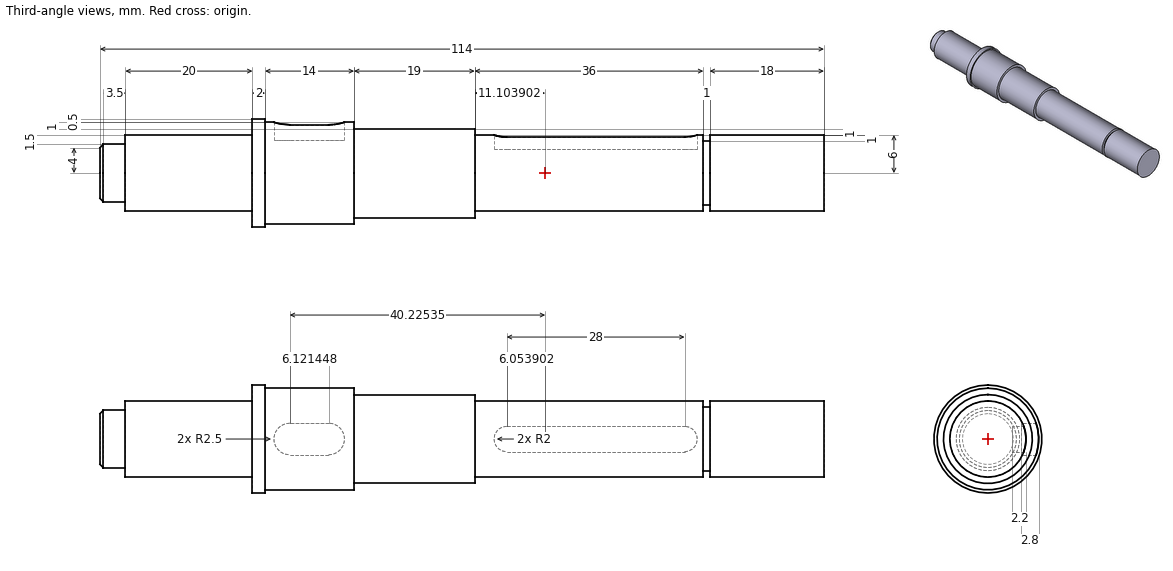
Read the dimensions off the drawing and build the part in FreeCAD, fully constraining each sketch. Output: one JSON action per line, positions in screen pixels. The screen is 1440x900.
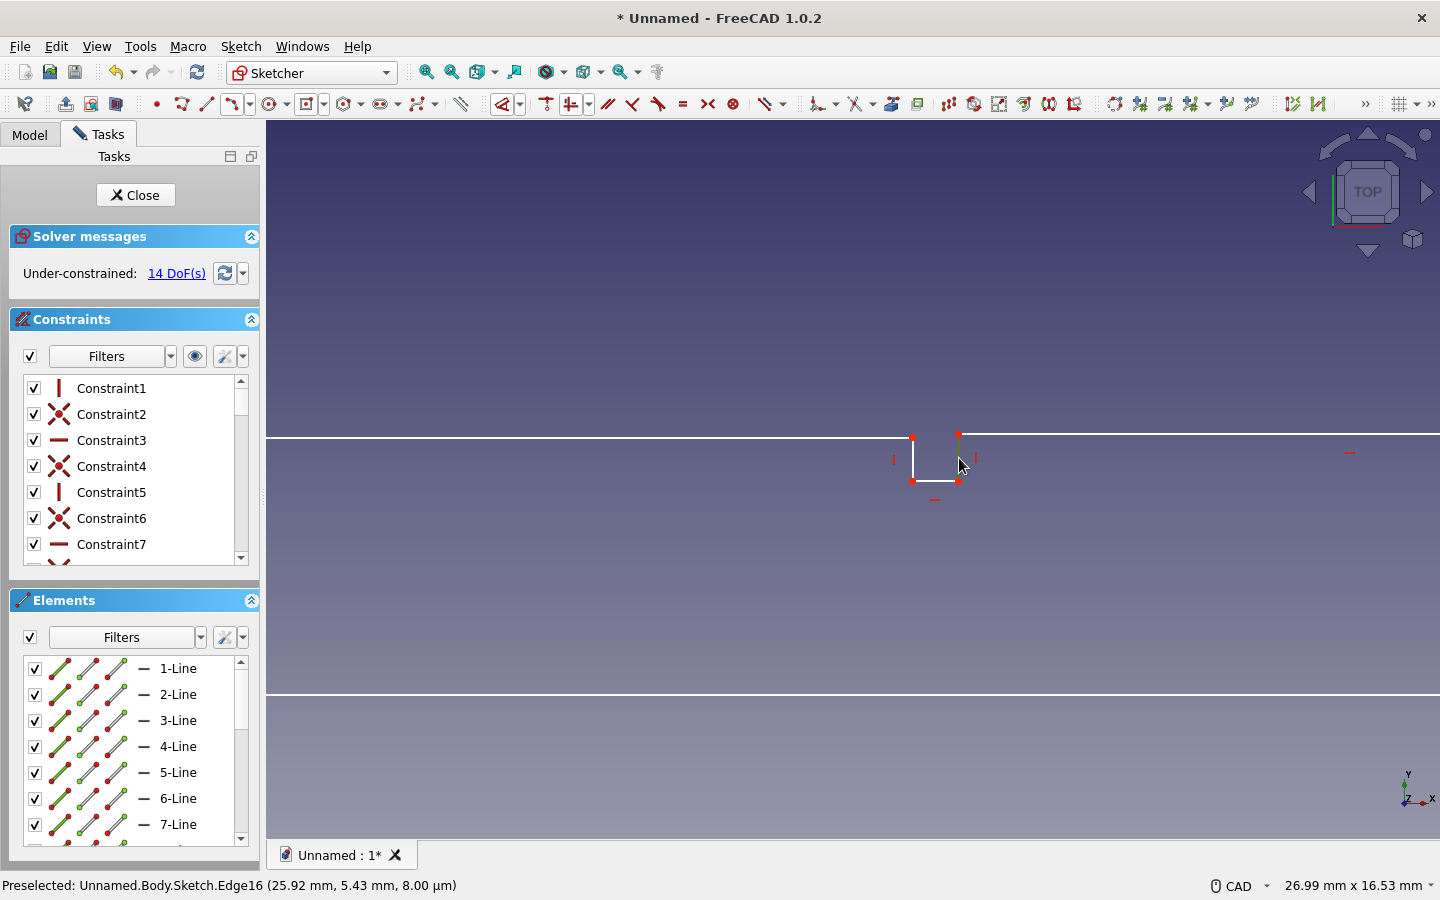
{"action": "left_click", "coordinate": [520, 104]}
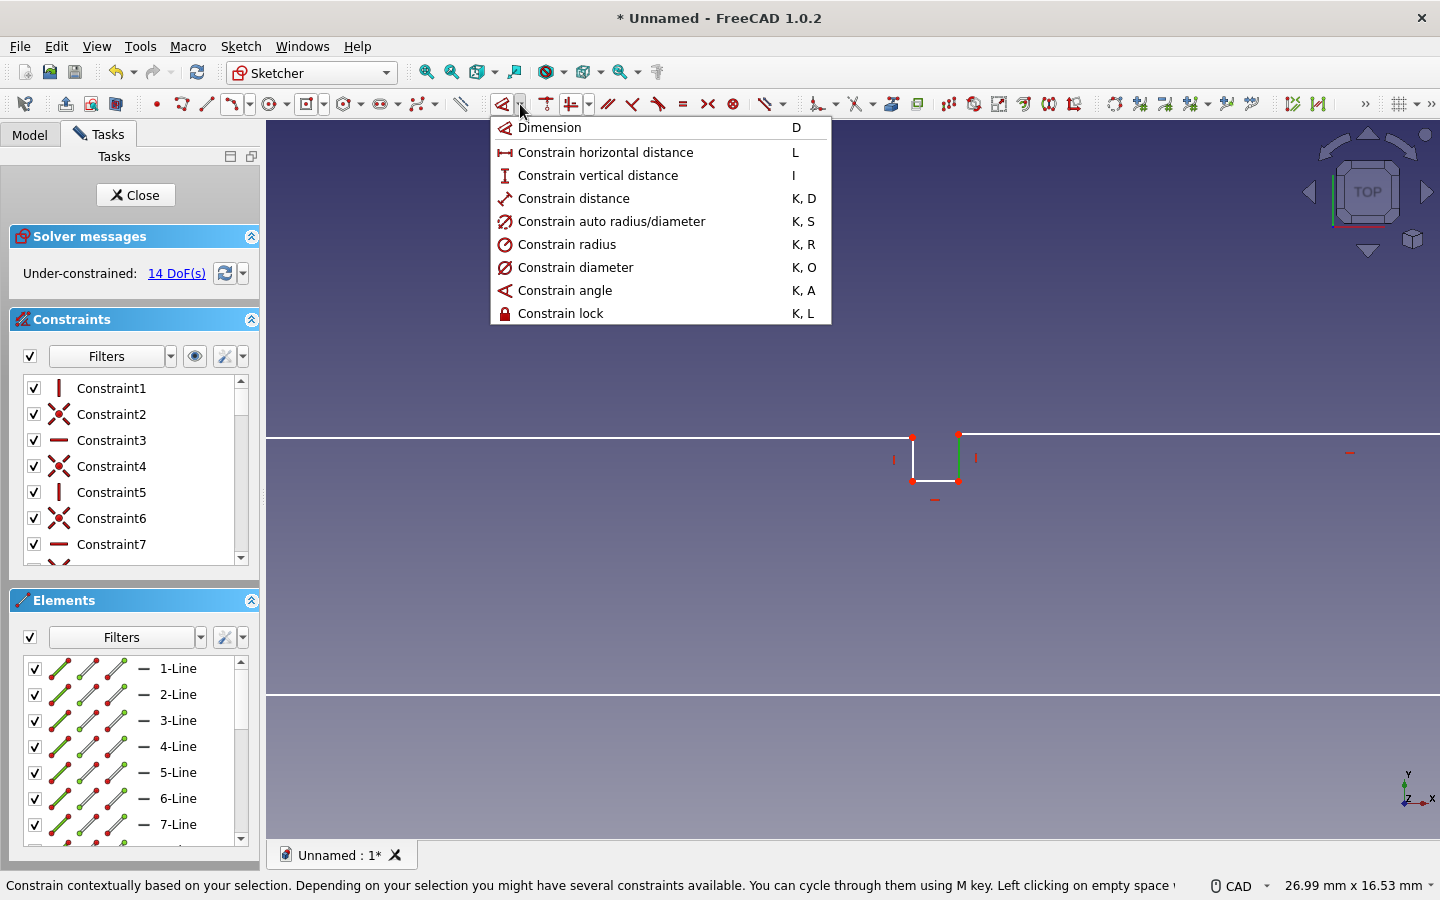
{"action": "left_click", "coordinate": [661, 176]}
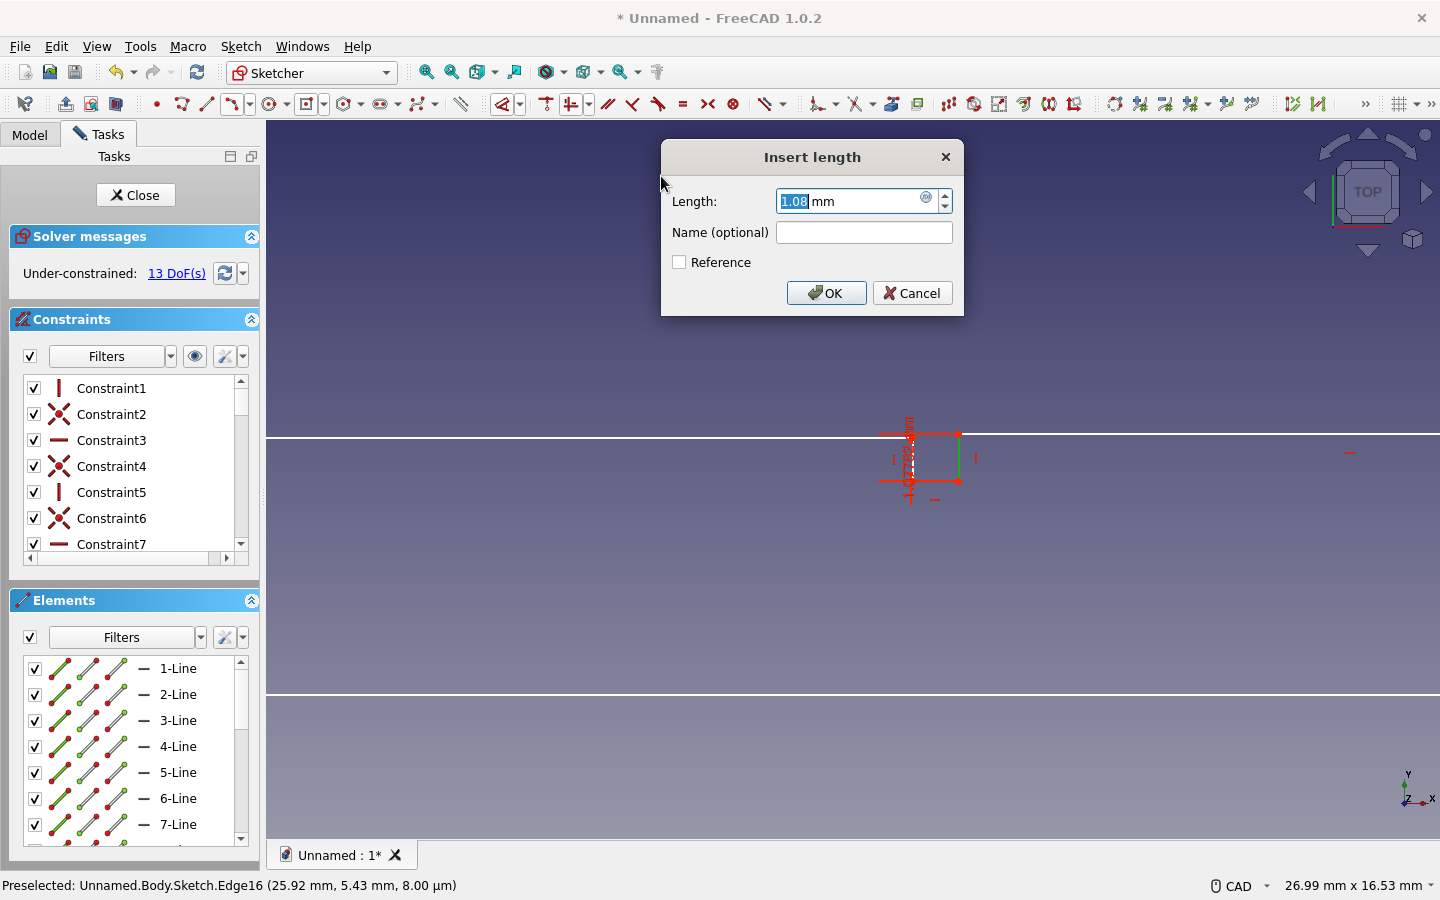
{"action": "type", "text": "1"}
{"action": "key", "text": "Return"}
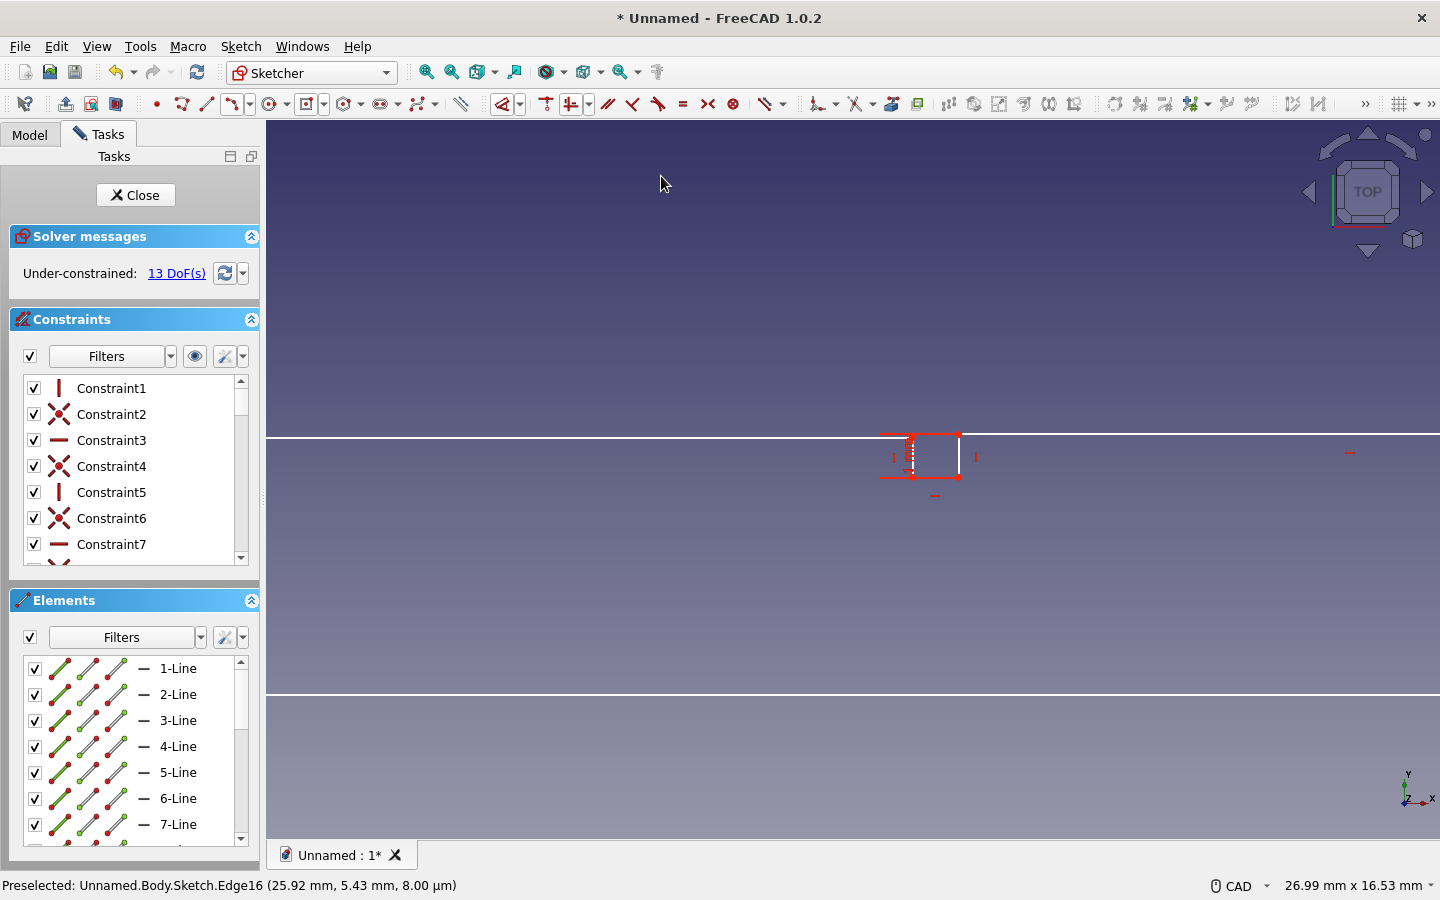
{"action": "left_click", "coordinate": [945, 478]}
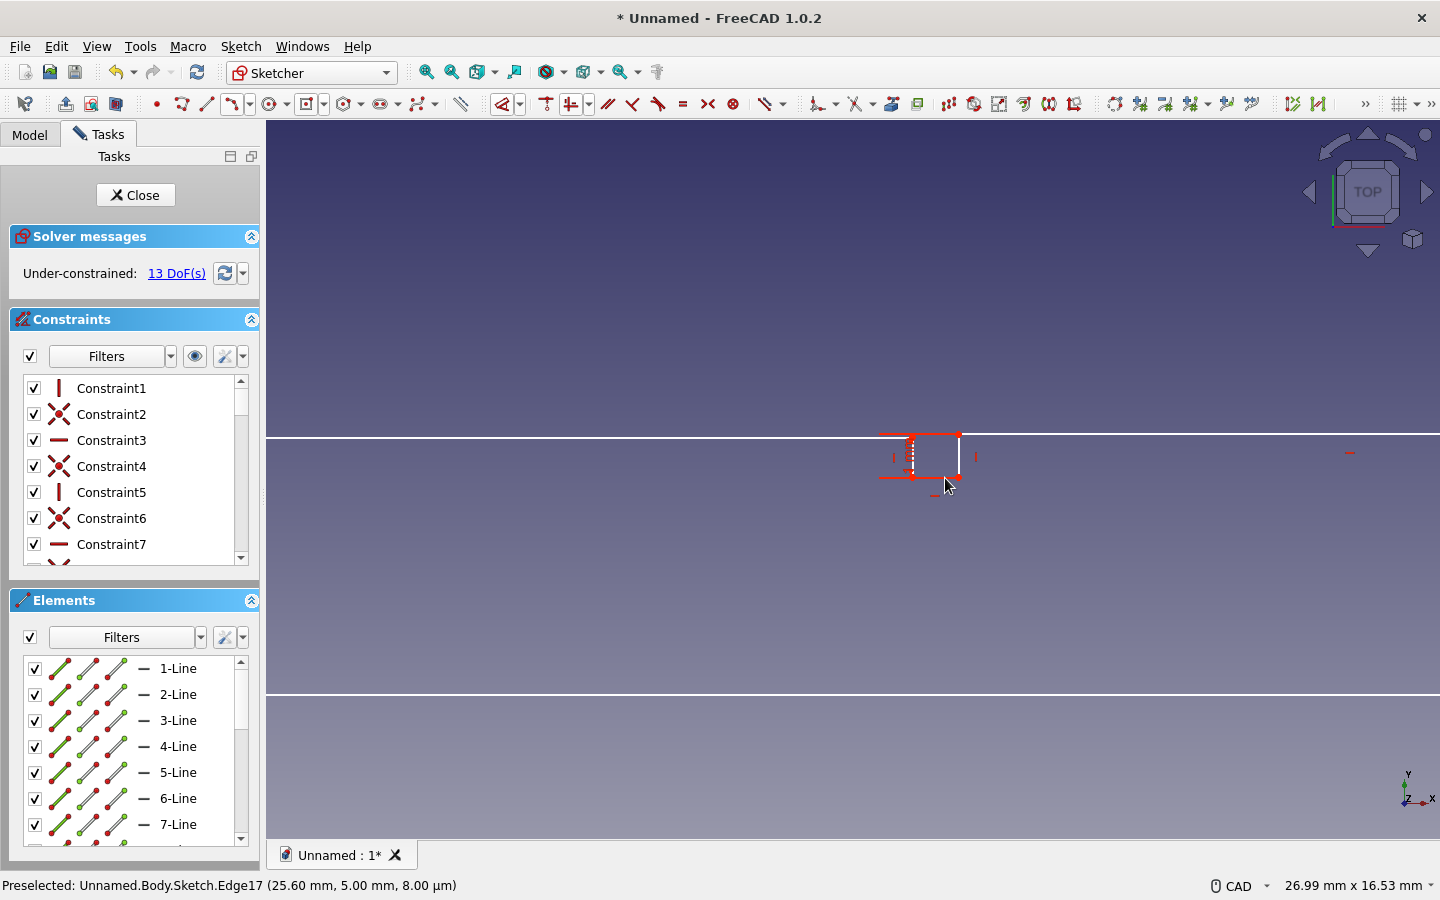
{"action": "left_click", "coordinate": [520, 104]}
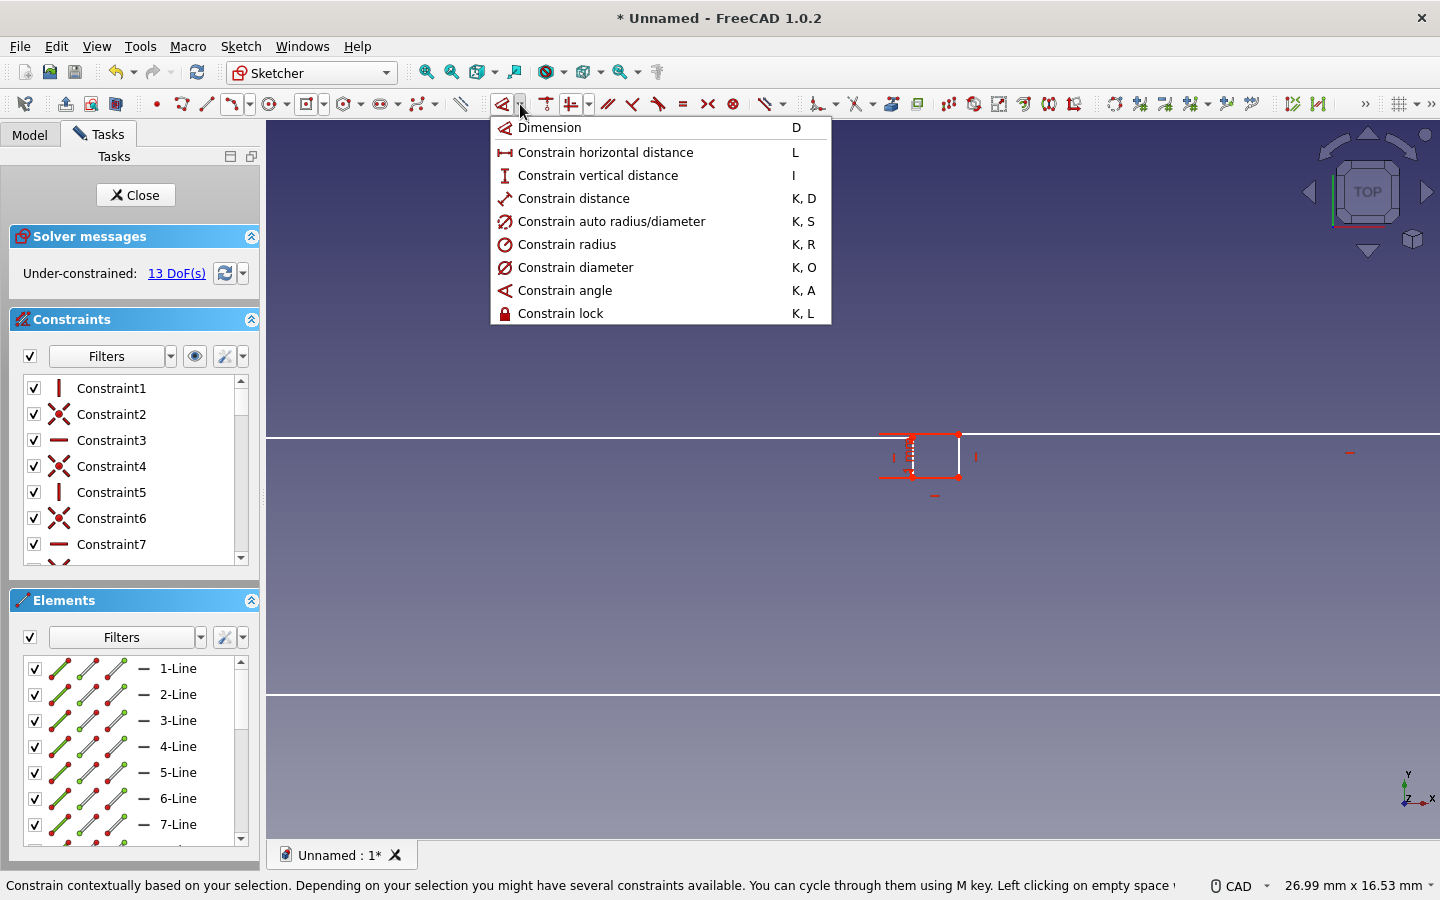
{"action": "left_click", "coordinate": [661, 152]}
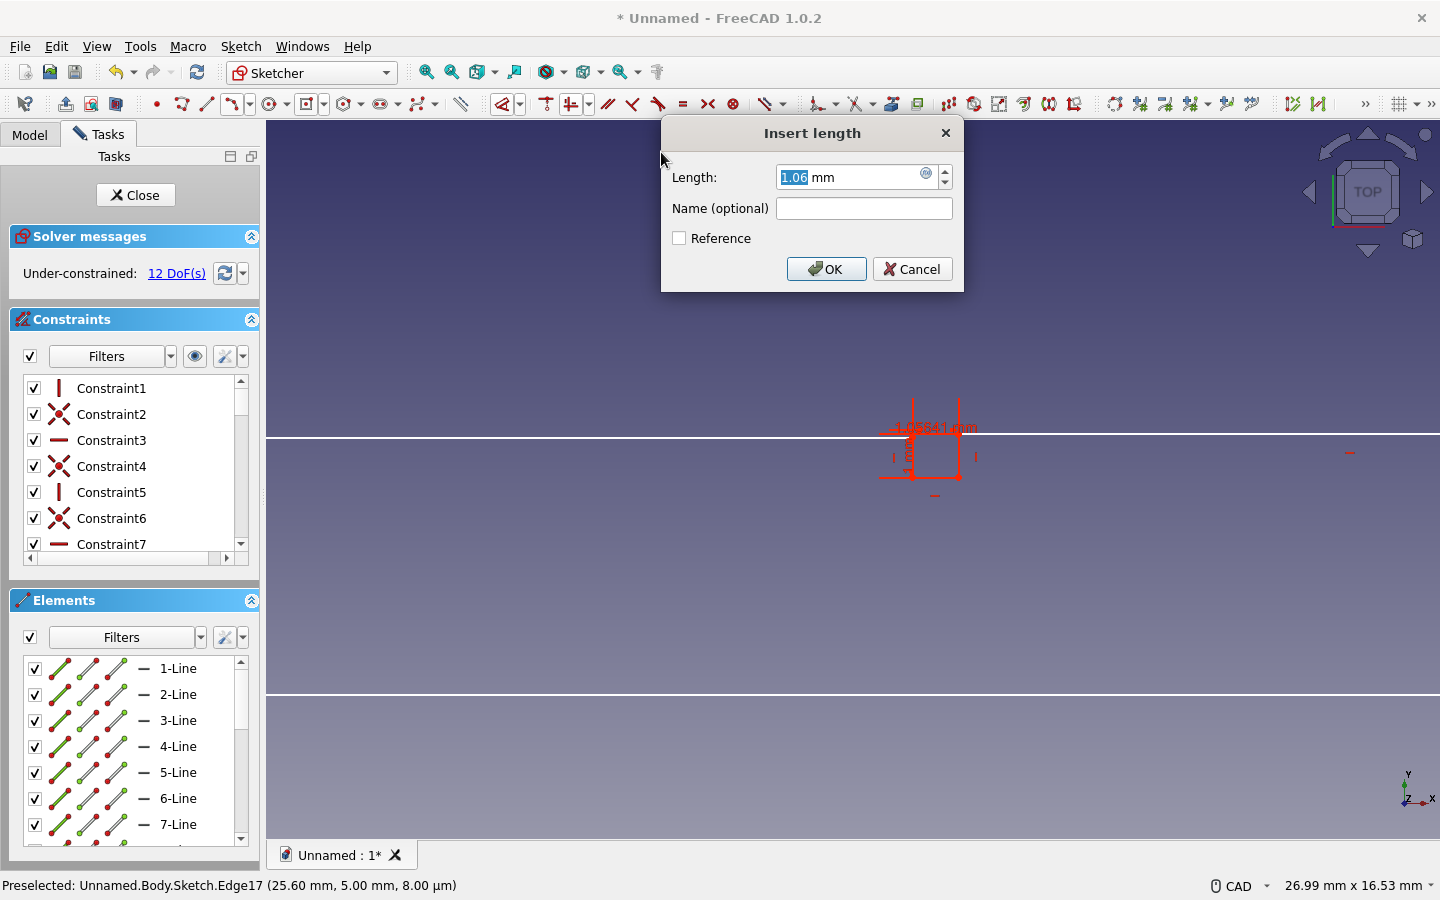
{"action": "type", "text": "1"}
{"action": "key", "text": "Return"}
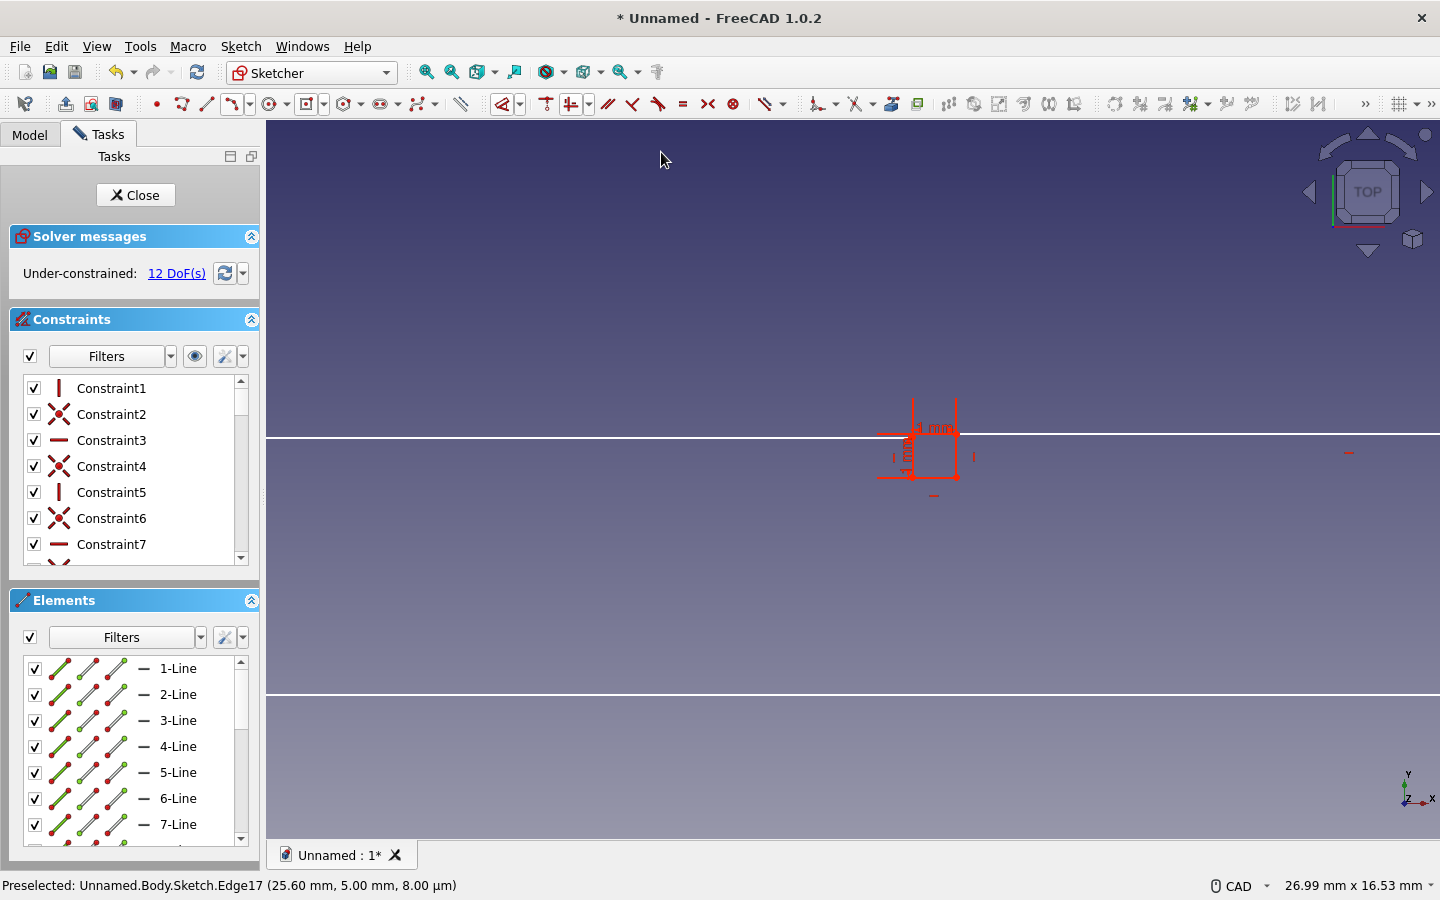
{"action": "scroll", "coordinate": [913, 466], "scroll_direction": "up", "scroll_amount": 4}